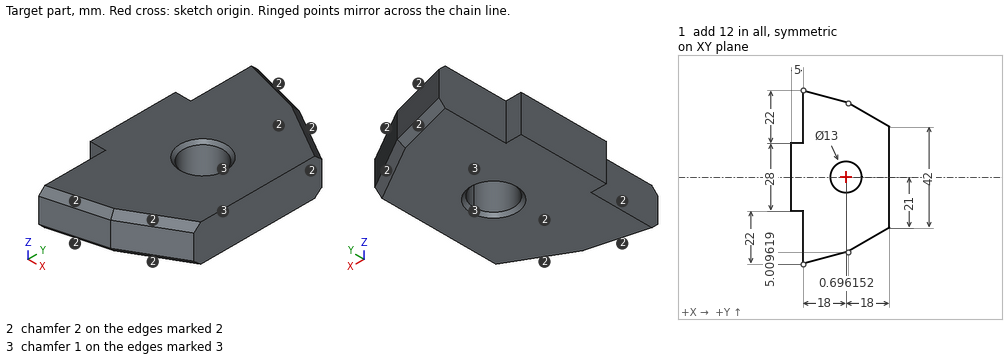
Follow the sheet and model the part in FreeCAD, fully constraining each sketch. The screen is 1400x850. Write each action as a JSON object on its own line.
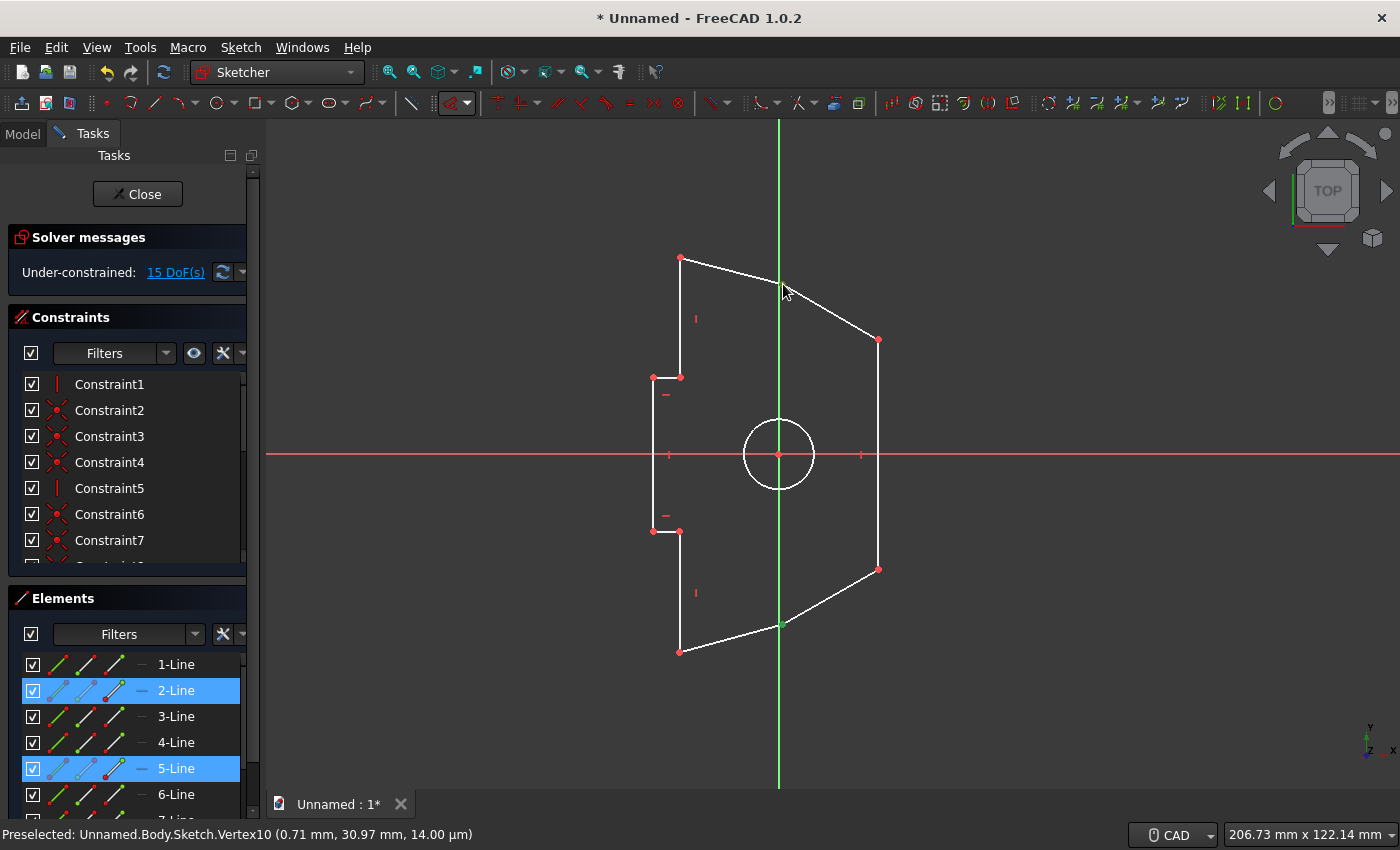
{"action": "left_click", "coordinate": [361, 454]}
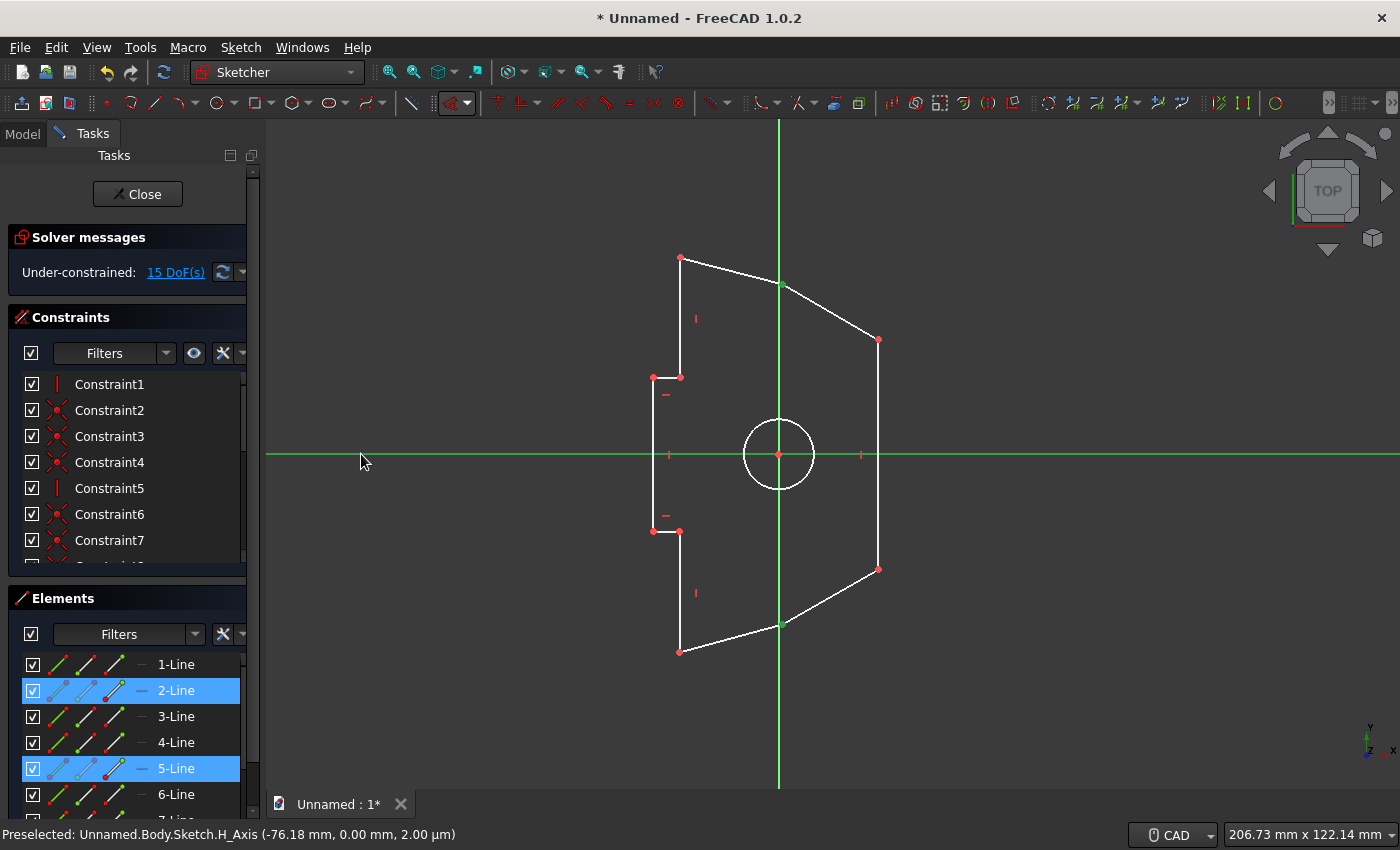
{"action": "left_click", "coordinate": [654, 104]}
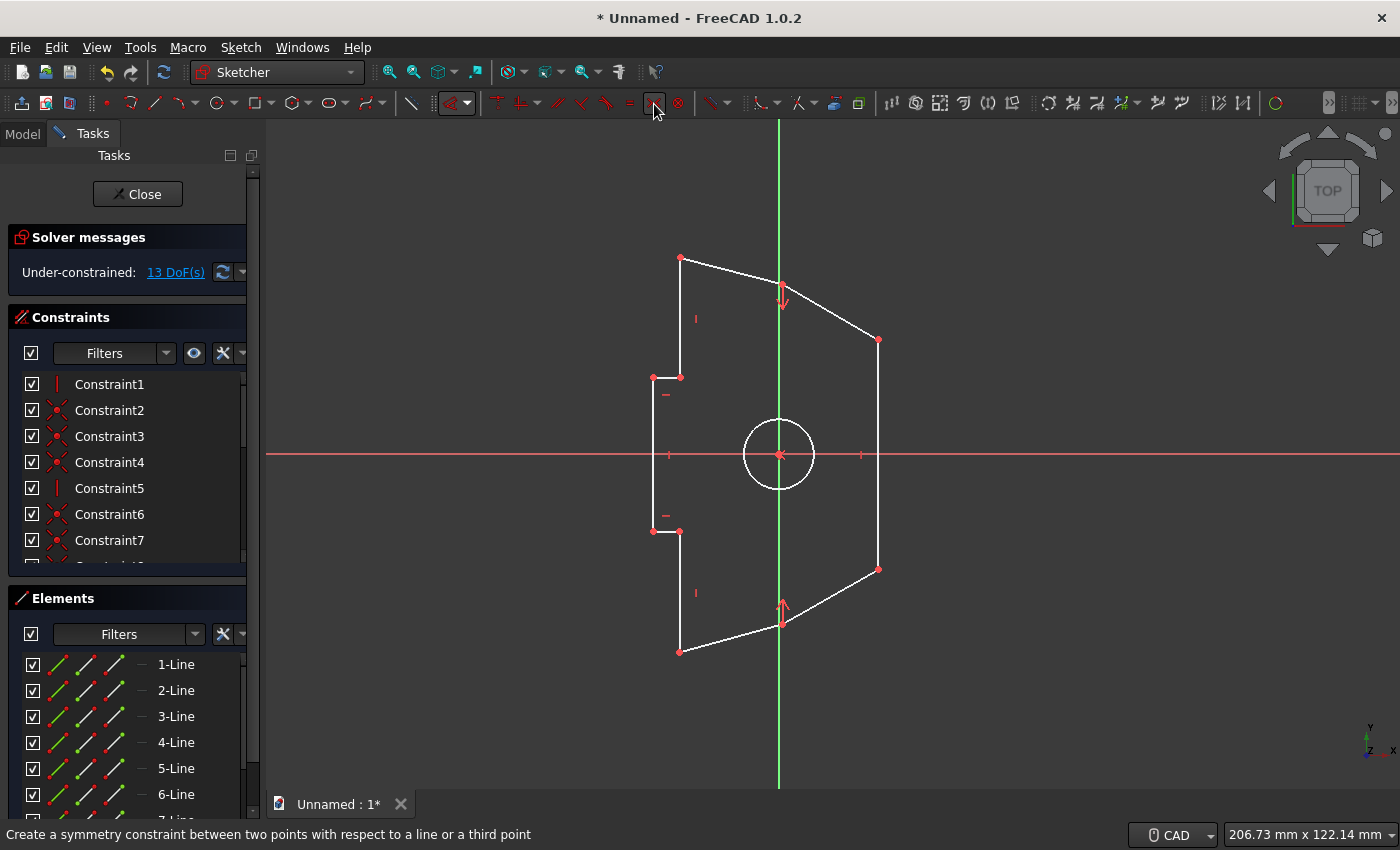
{"action": "left_click", "coordinate": [680, 652]}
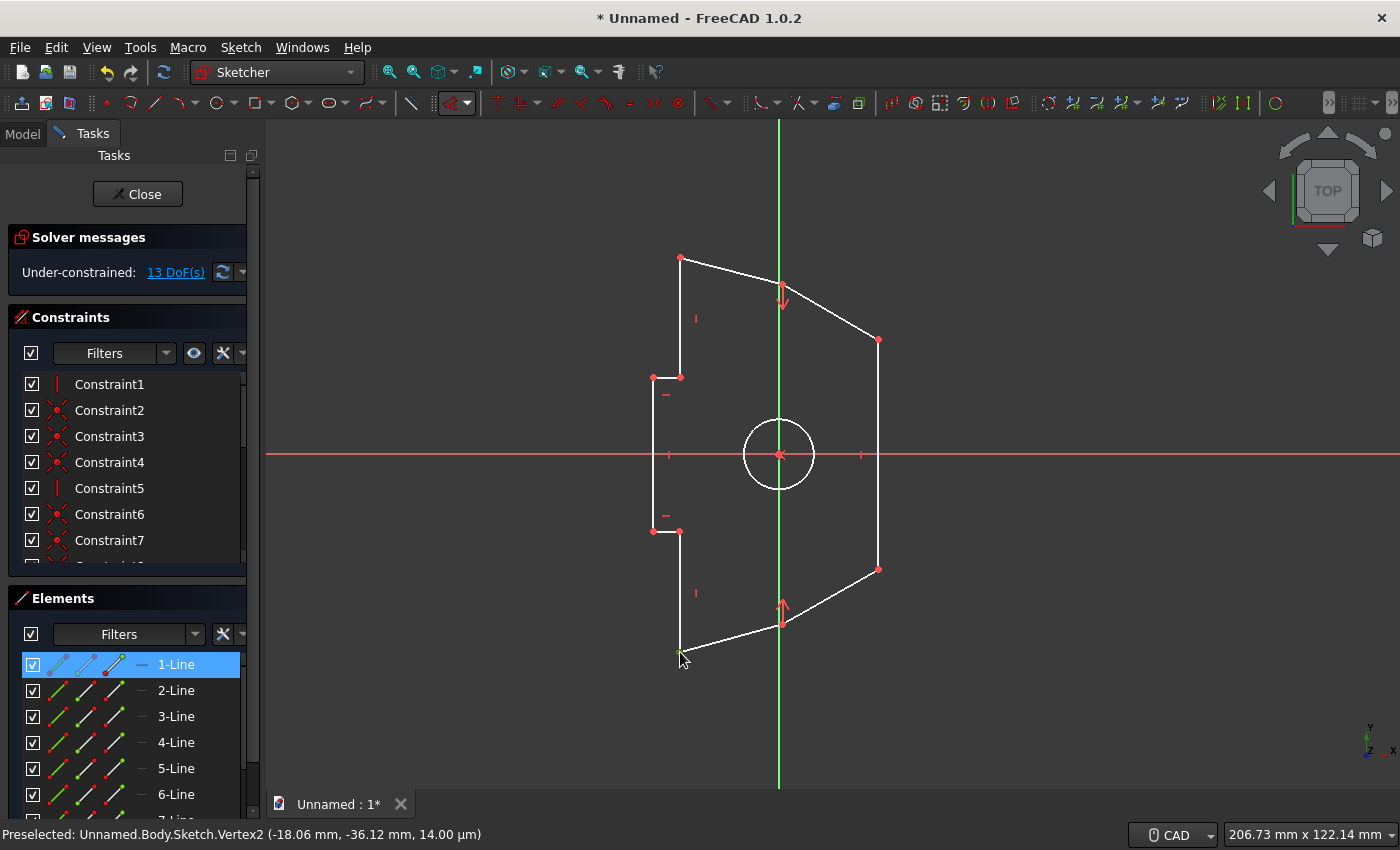
{"action": "left_click", "coordinate": [680, 258]}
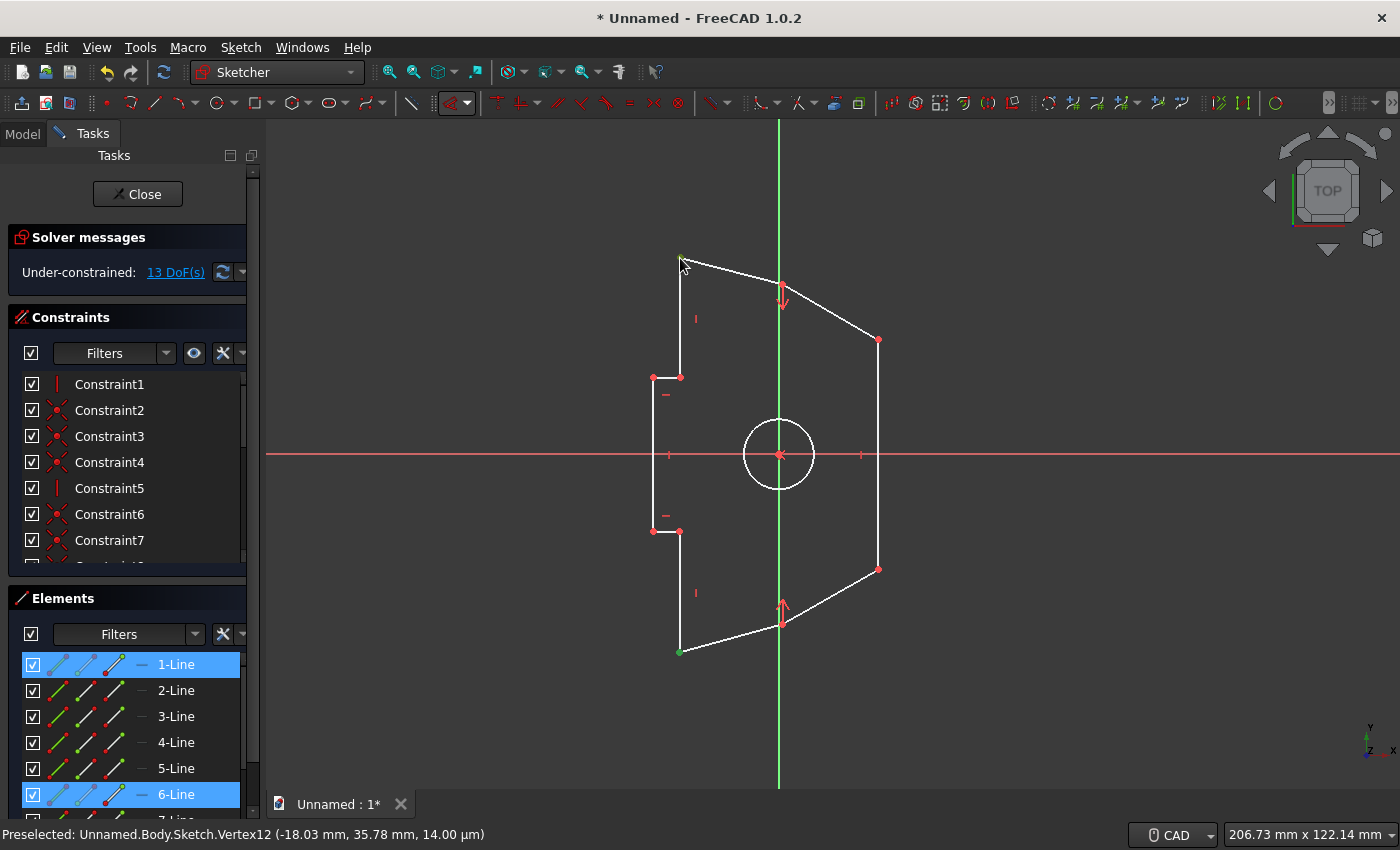
{"action": "left_click", "coordinate": [361, 454]}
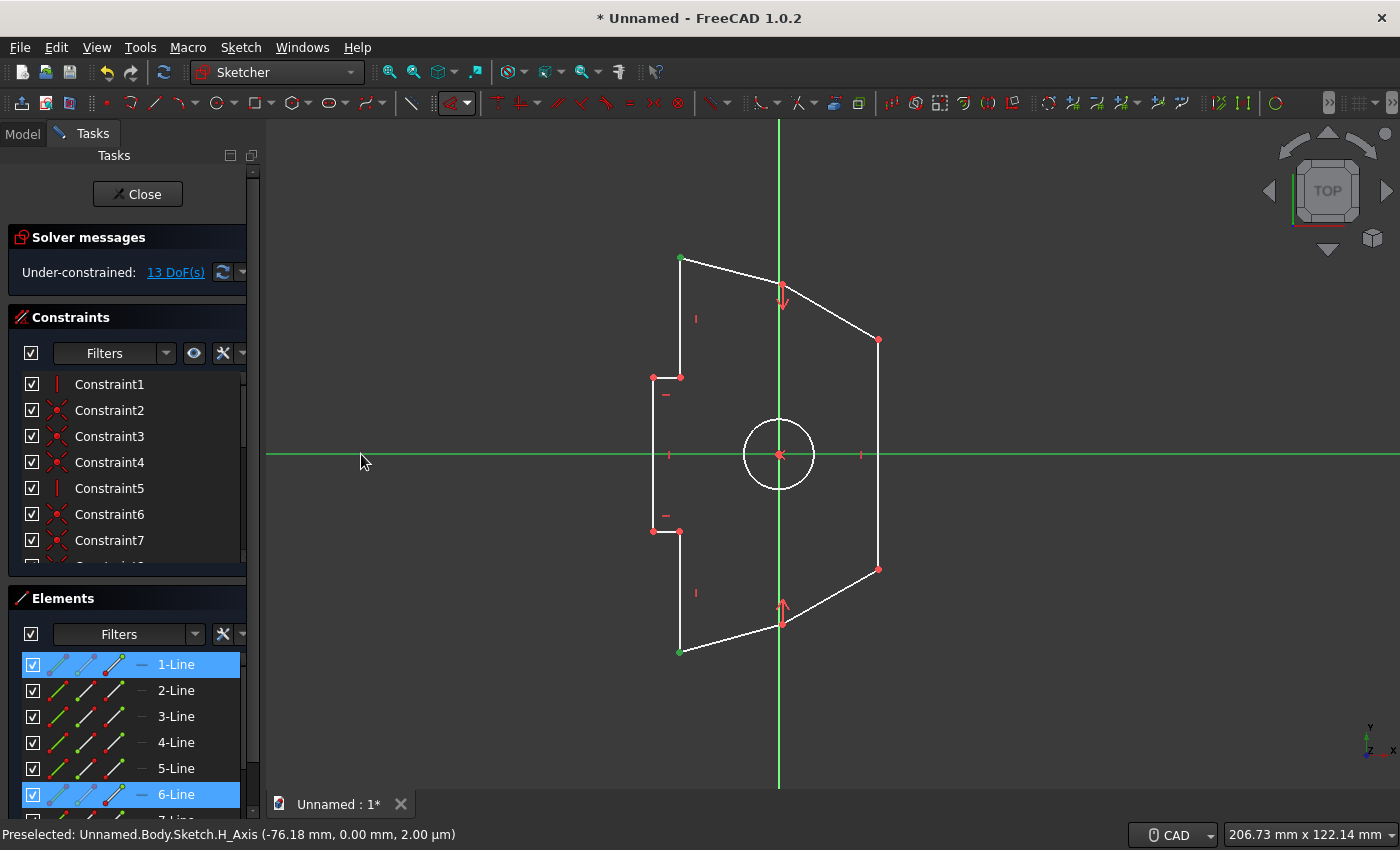
{"action": "left_click", "coordinate": [654, 104]}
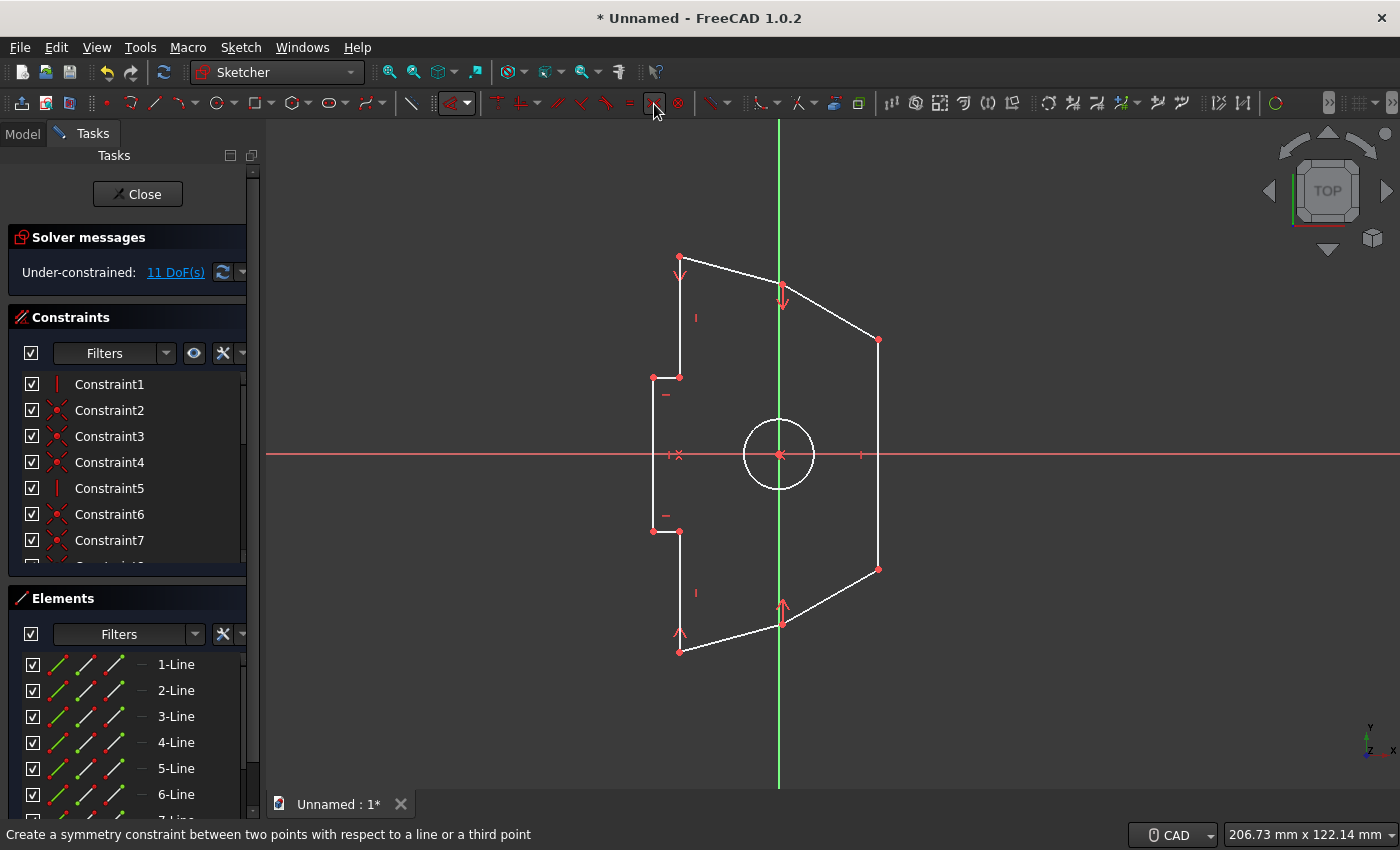
{"action": "left_click", "coordinate": [450, 104]}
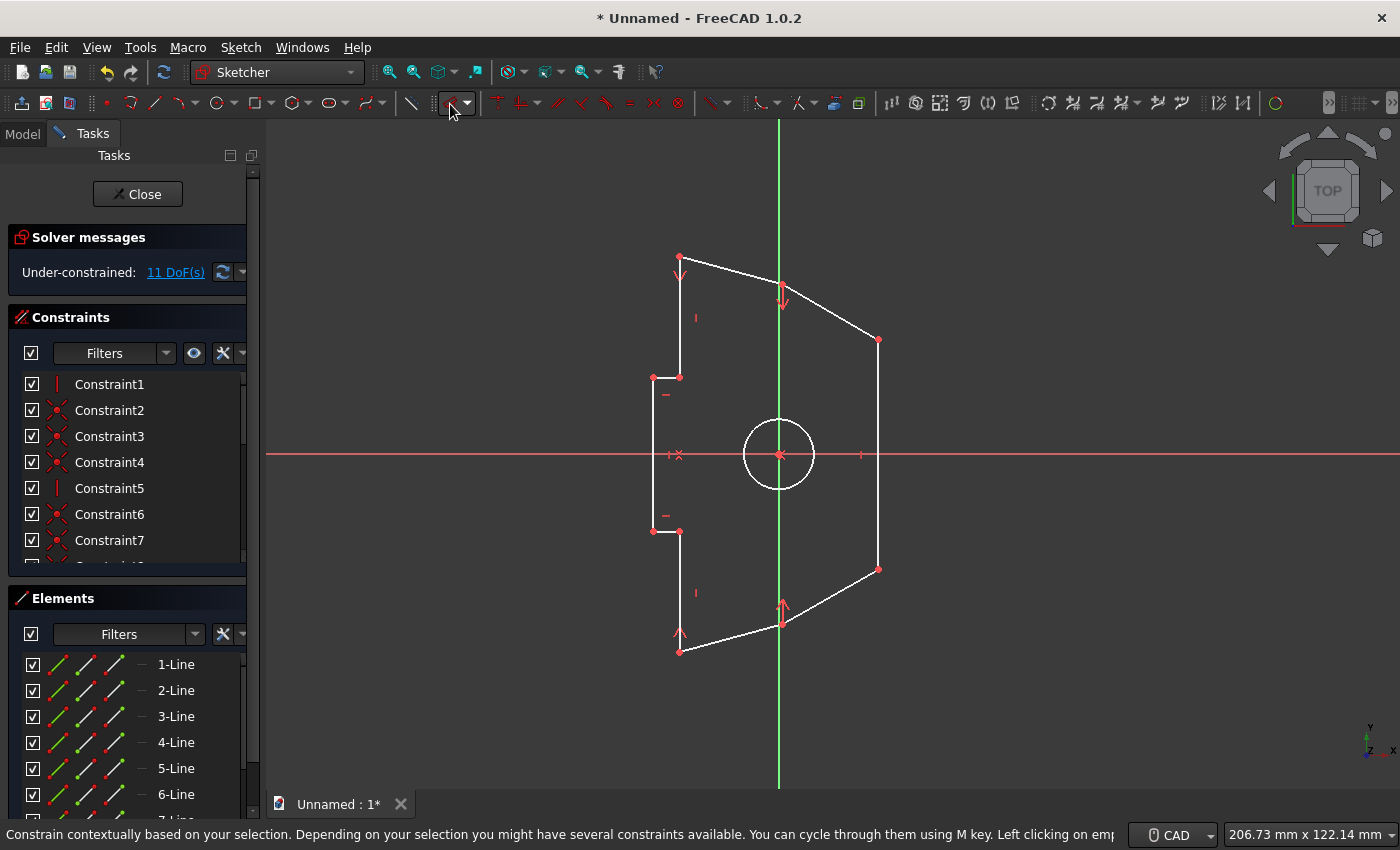
{"action": "left_click", "coordinate": [804, 430]}
{"action": "left_click", "coordinate": [827, 408]}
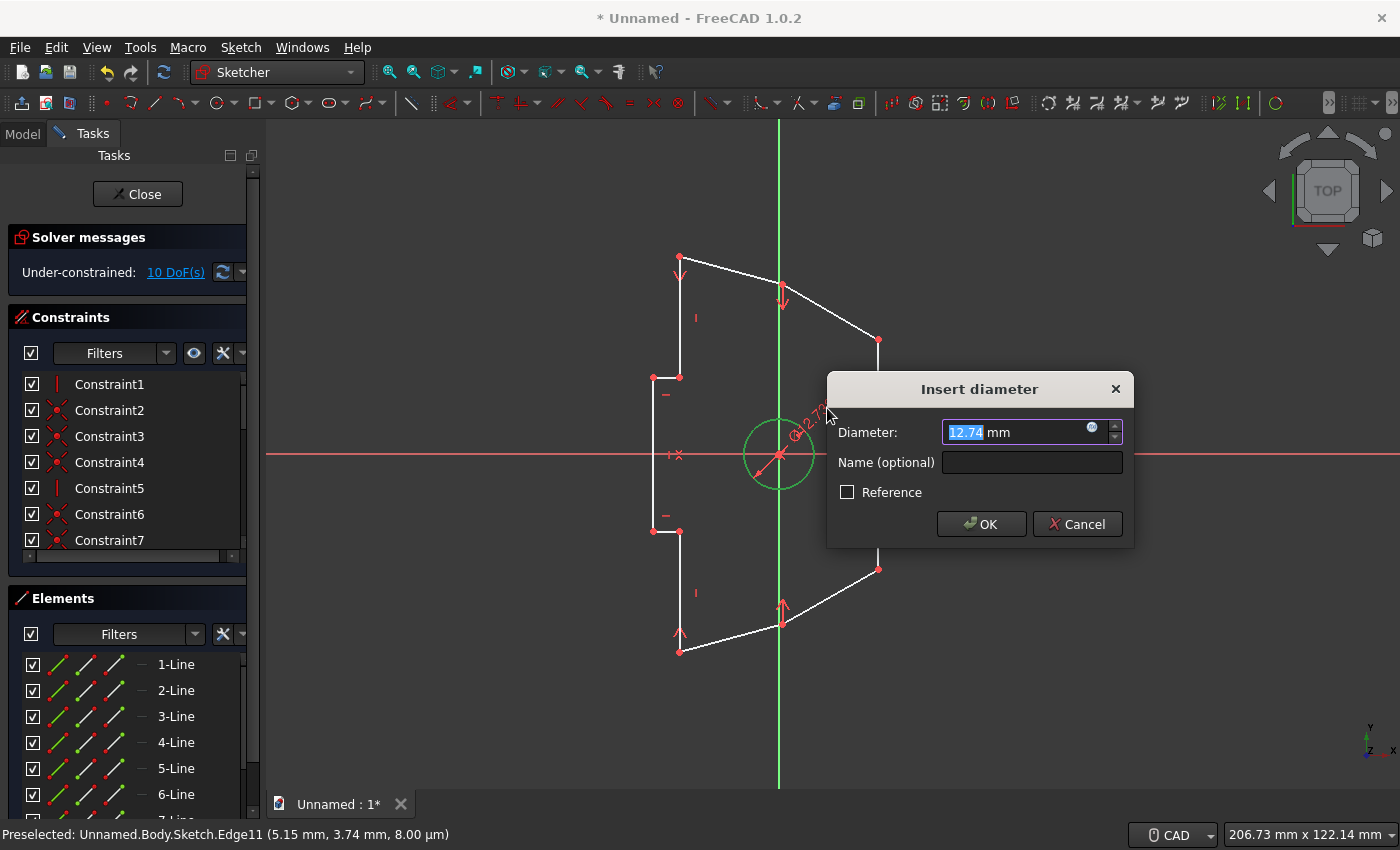
{"action": "type", "text": "13"}
{"action": "key", "text": "Return"}